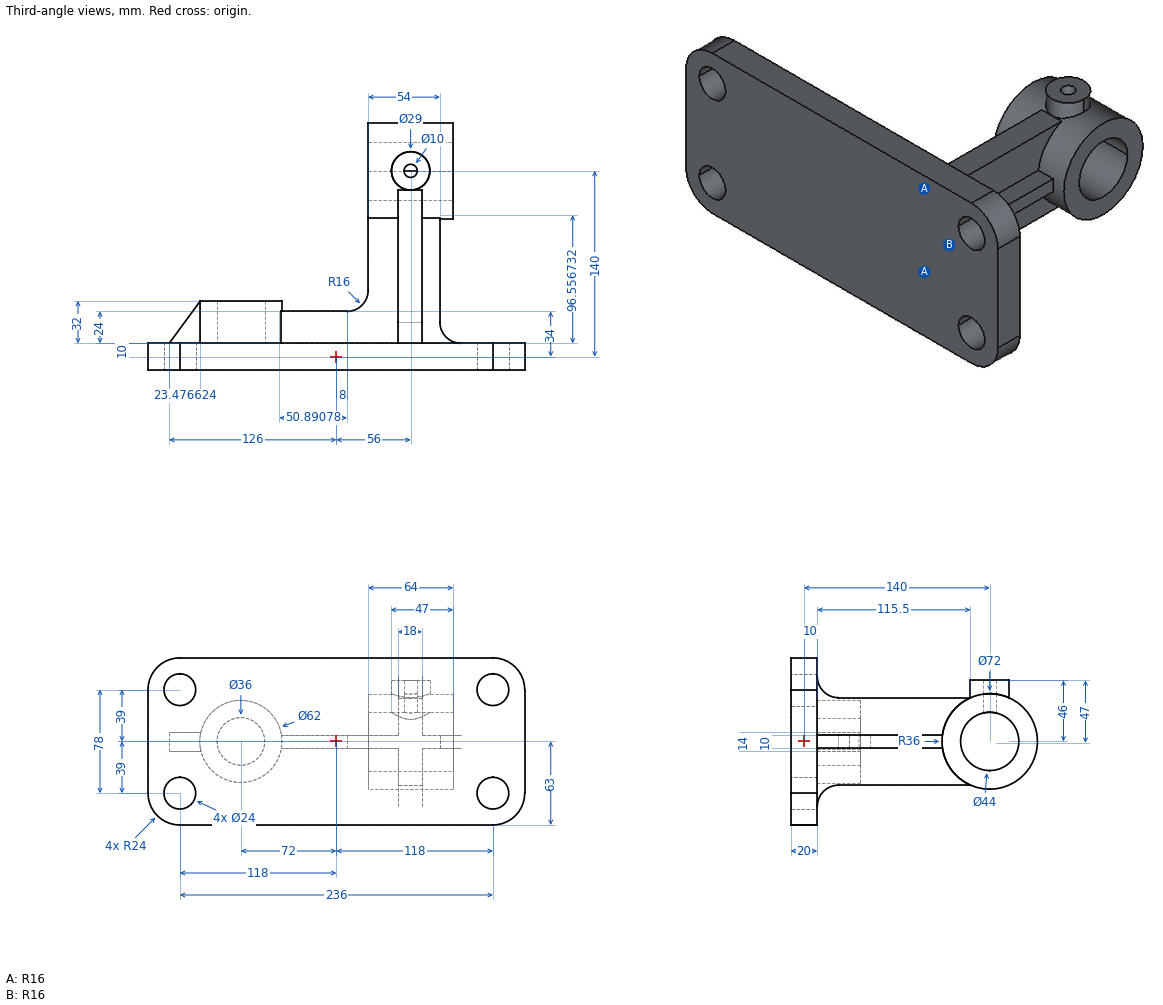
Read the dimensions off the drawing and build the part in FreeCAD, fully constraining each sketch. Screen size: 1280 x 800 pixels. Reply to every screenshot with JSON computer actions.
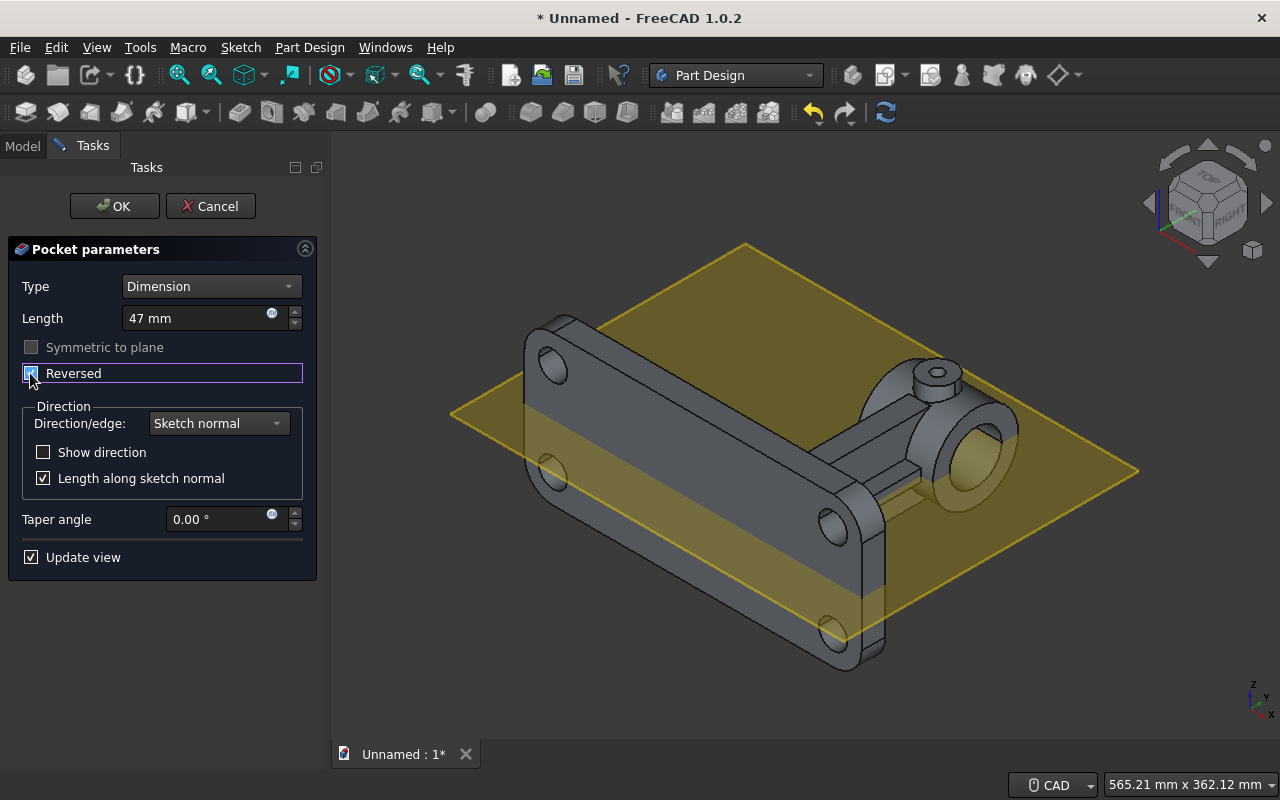
{"action": "left_click", "coordinate": [115, 206]}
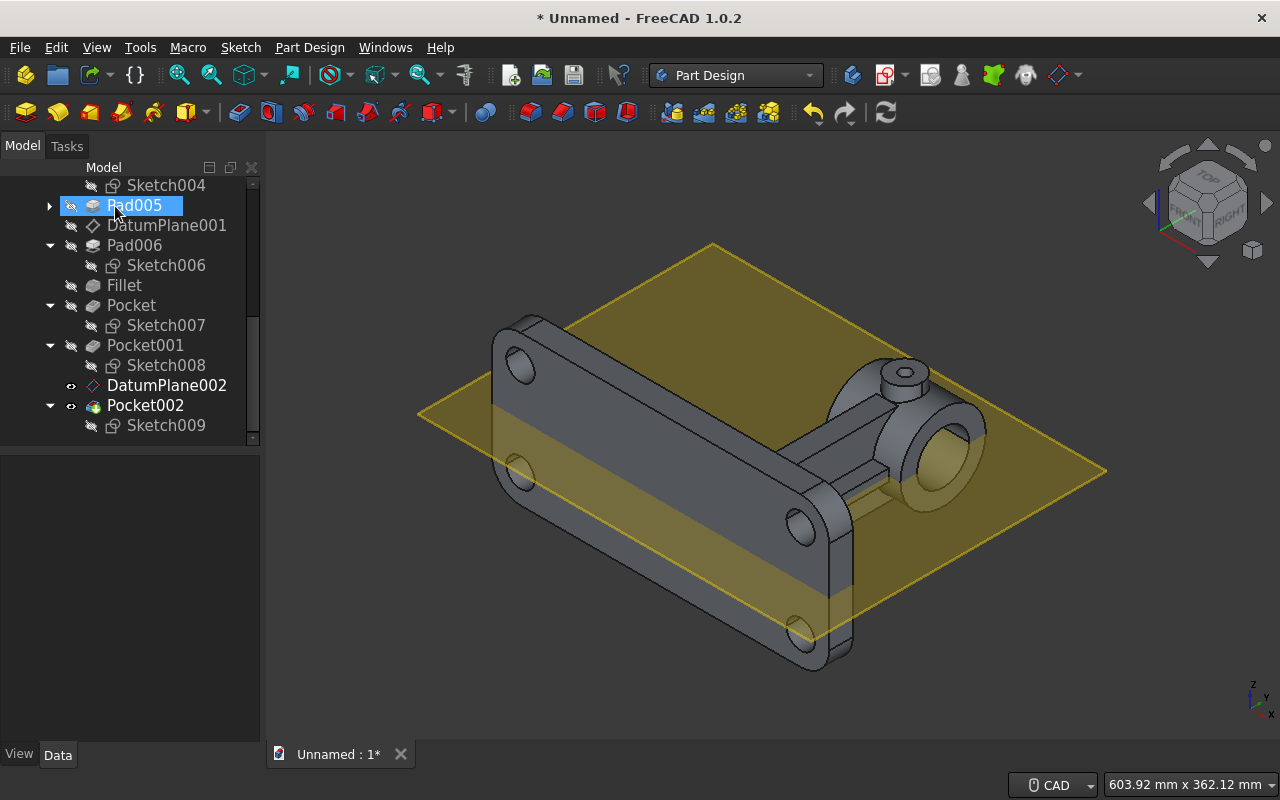
{"action": "left_click", "coordinate": [116, 386]}
{"action": "key", "text": "space"}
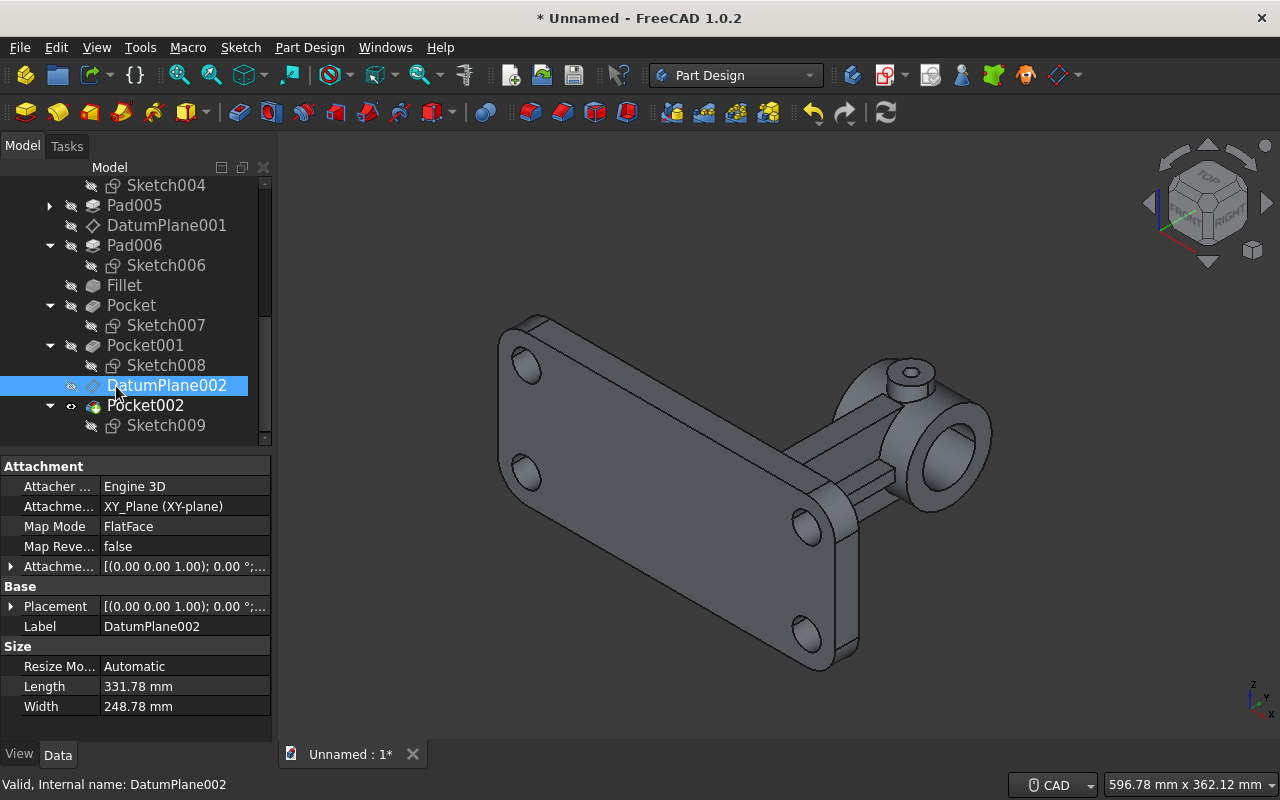
{"action": "scroll", "coordinate": [783, 539], "scroll_direction": "up", "scroll_amount": 5}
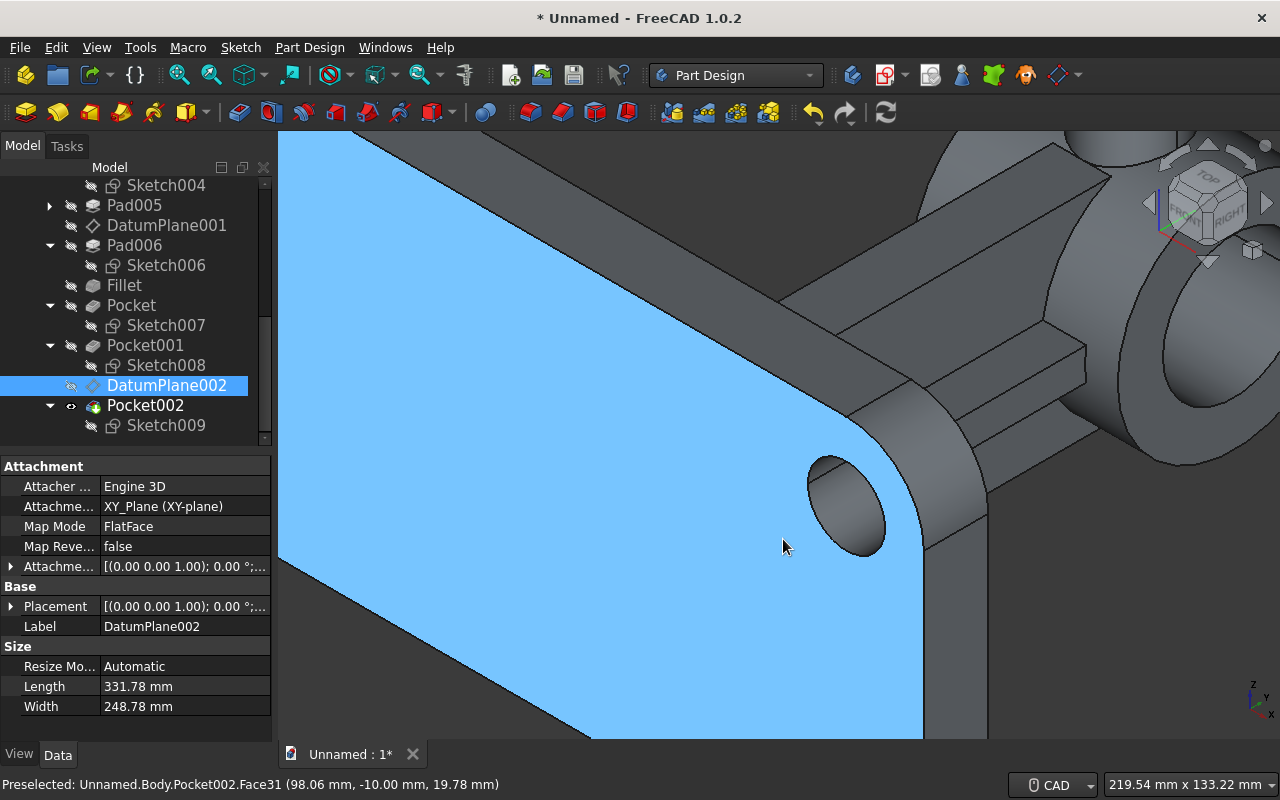
{"action": "left_click", "coordinate": [180, 76]}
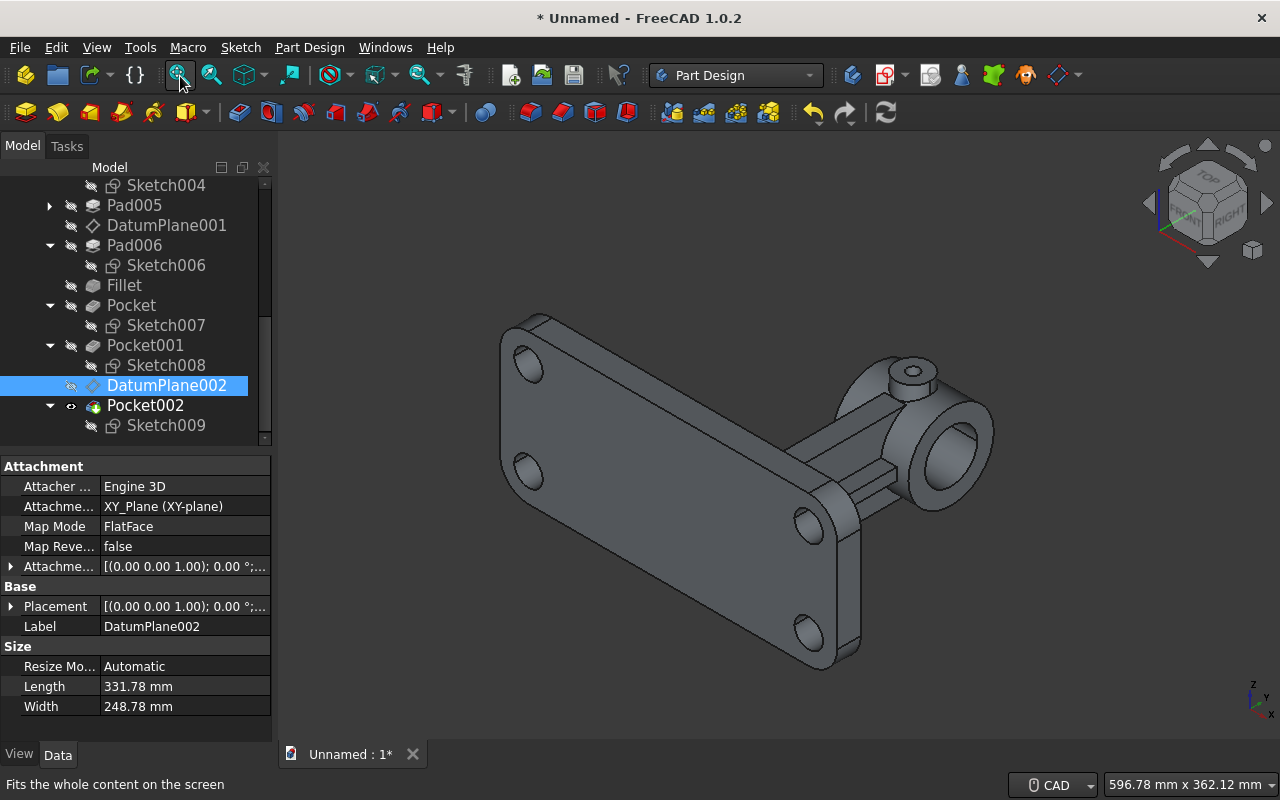
{"action": "key", "text": "2"}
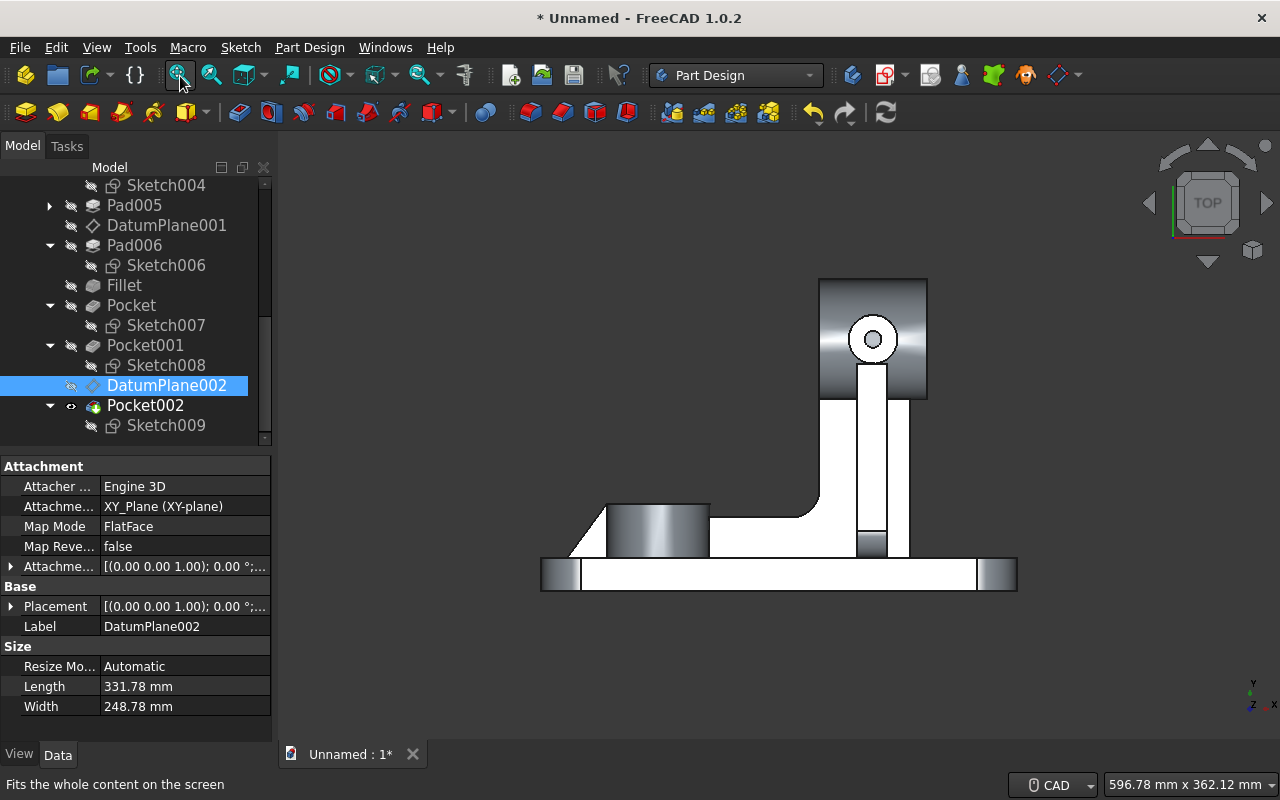
{"action": "scroll", "coordinate": [910, 557], "scroll_direction": "up", "scroll_amount": 5}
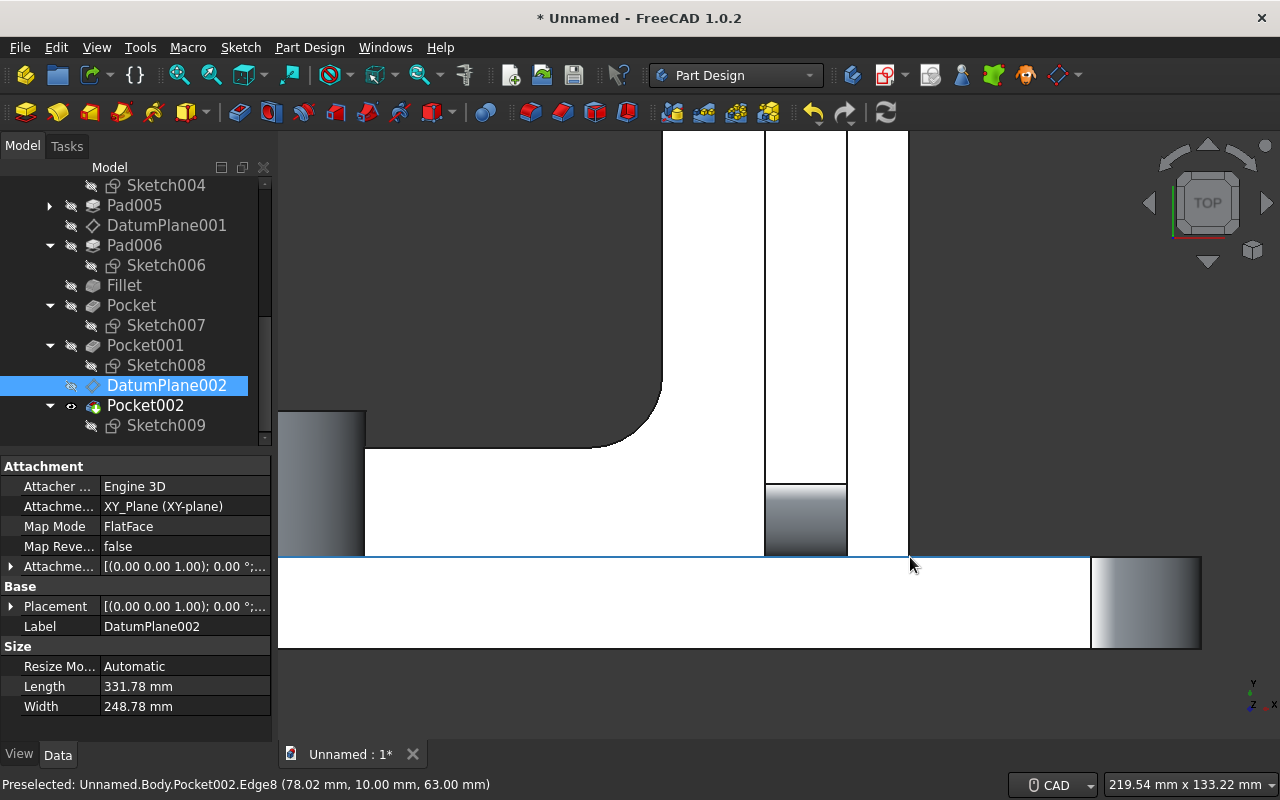
{"action": "left_click", "coordinate": [180, 76]}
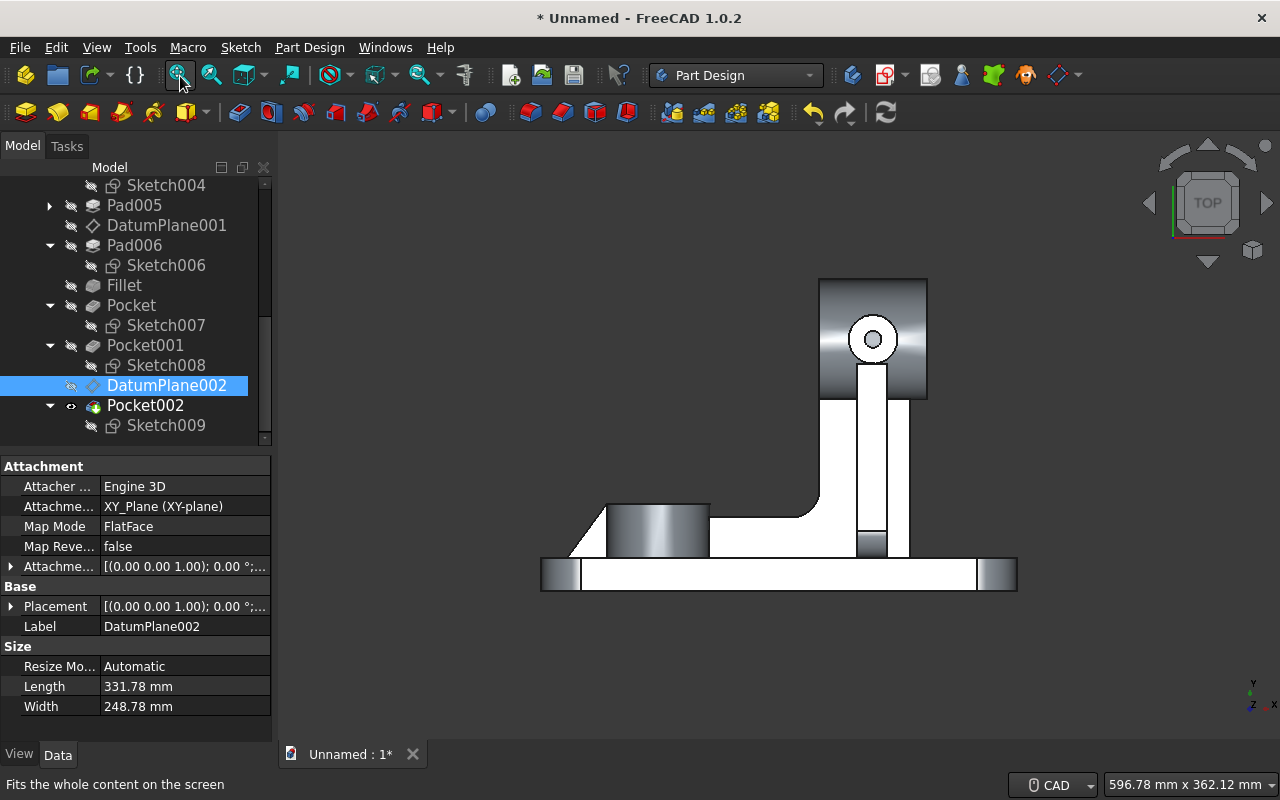
{"action": "key", "text": "0"}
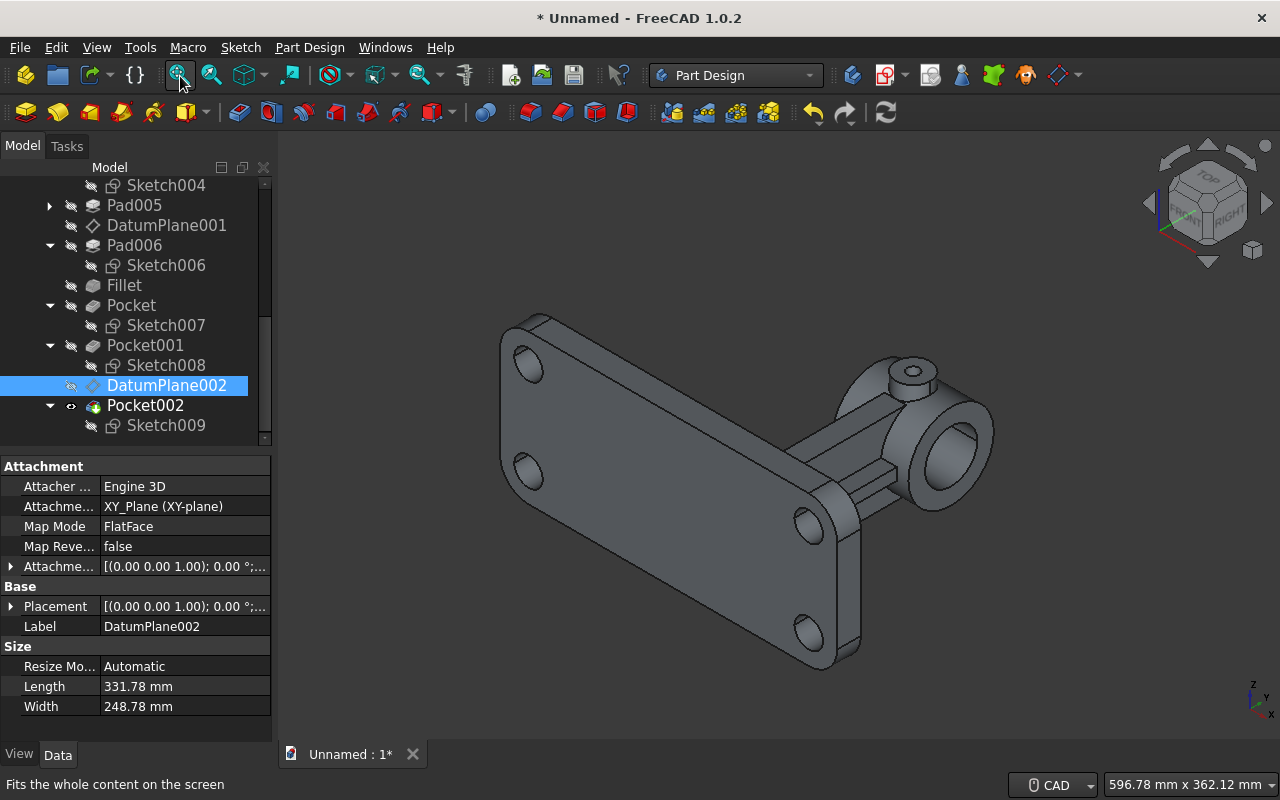
{"action": "scroll", "coordinate": [785, 538], "scroll_direction": "up", "scroll_amount": 5}